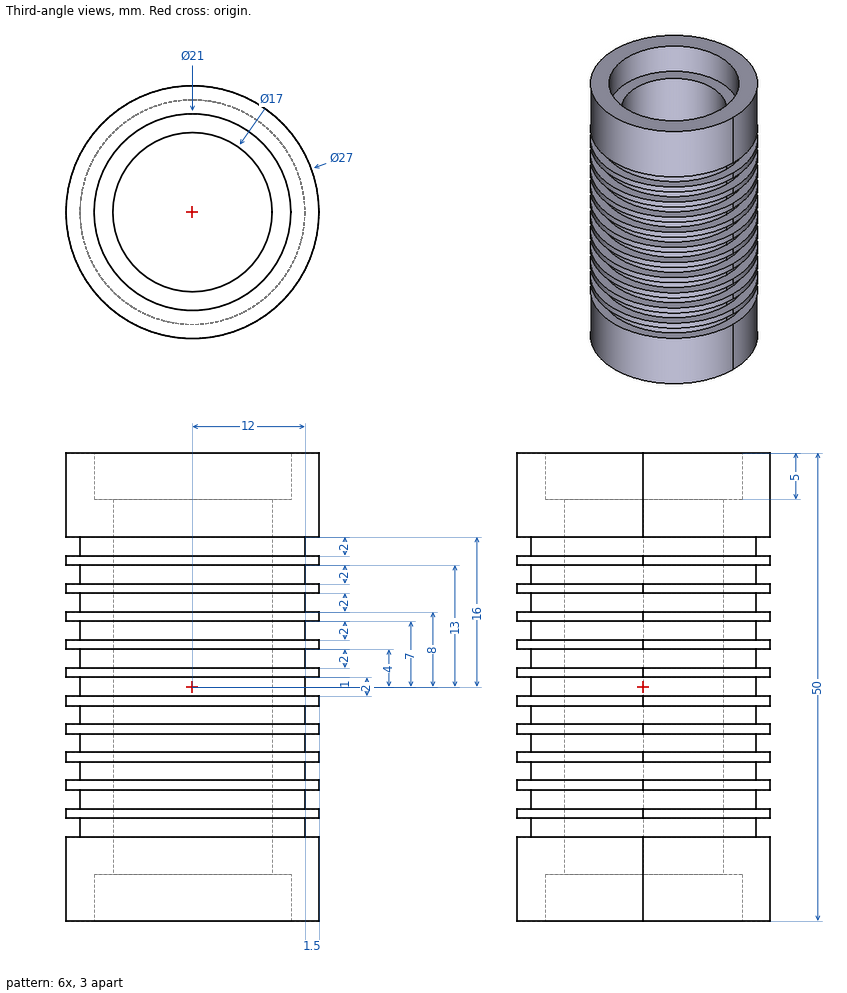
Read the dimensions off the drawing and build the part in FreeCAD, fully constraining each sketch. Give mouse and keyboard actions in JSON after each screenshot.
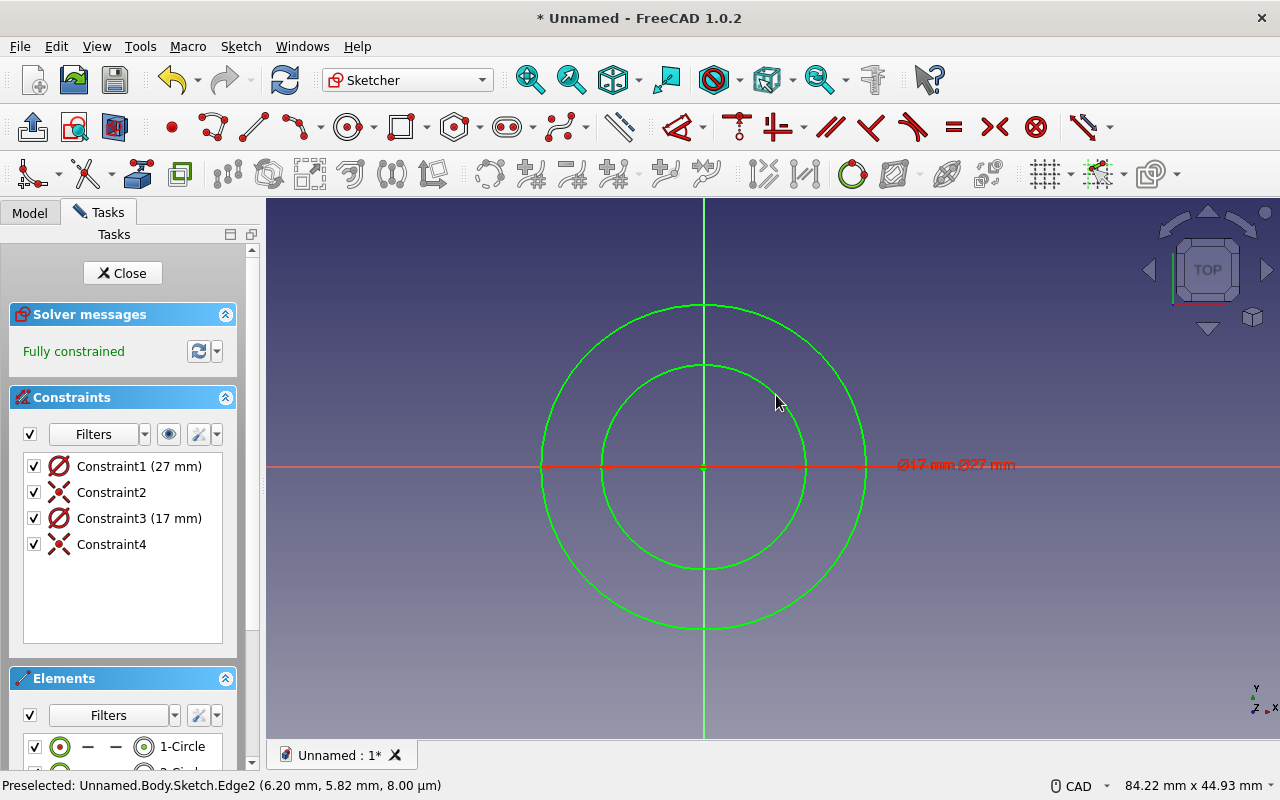
{"action": "left_click", "coordinate": [123, 273]}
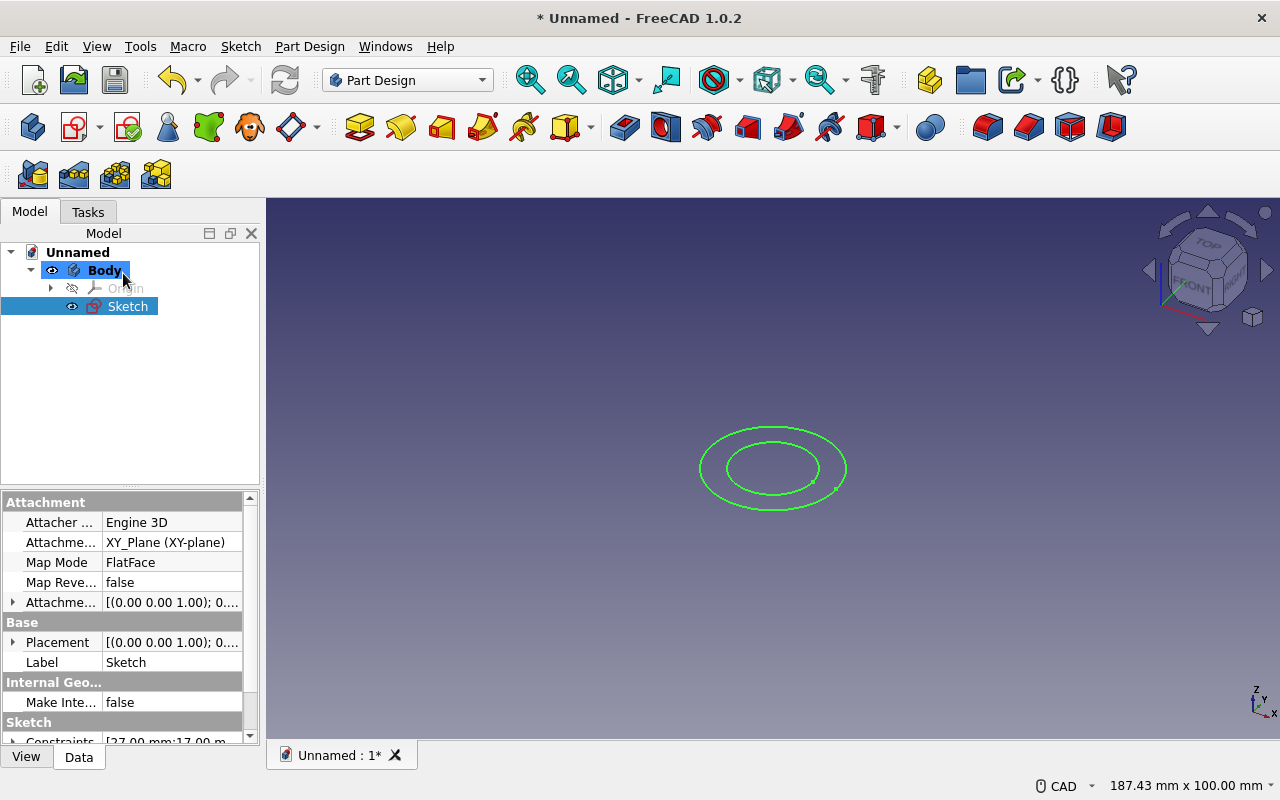
{"action": "left_click", "coordinate": [360, 128]}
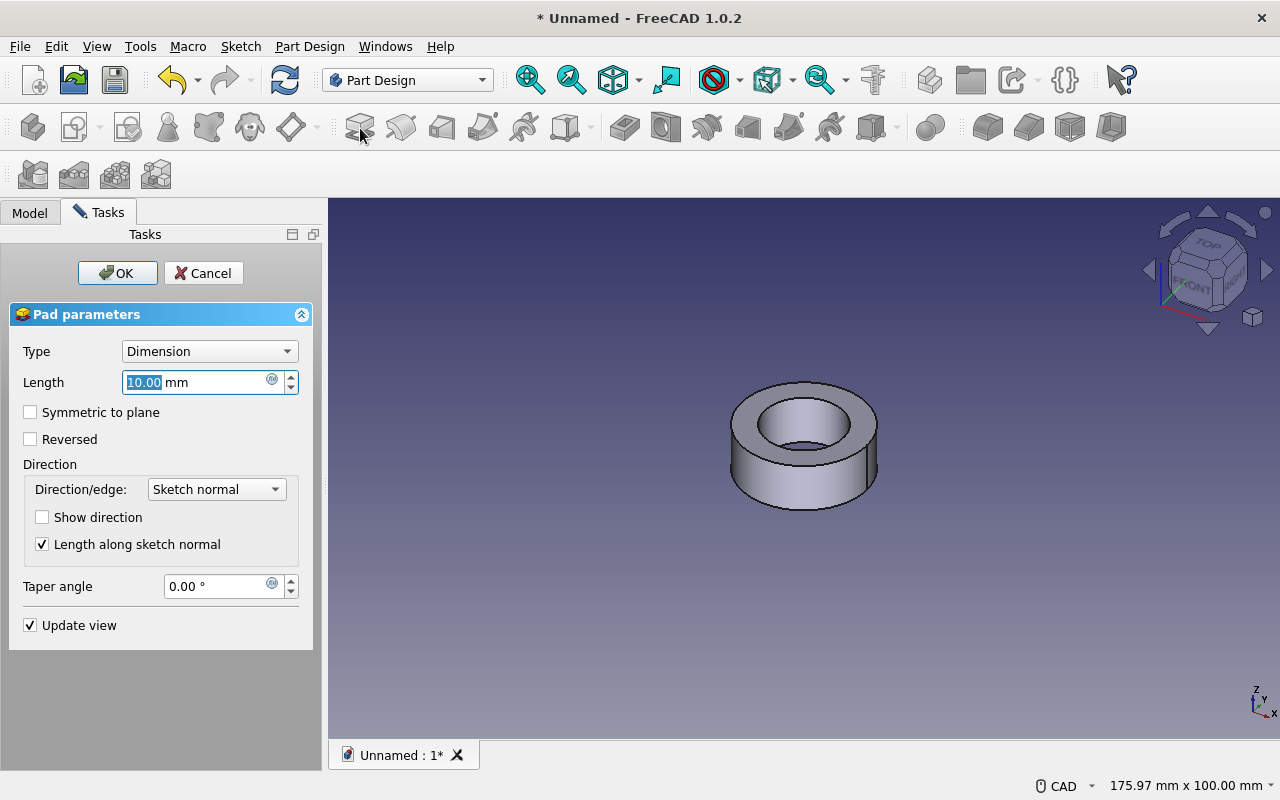
{"action": "type", "text": "50"}
{"action": "key", "text": "Tab"}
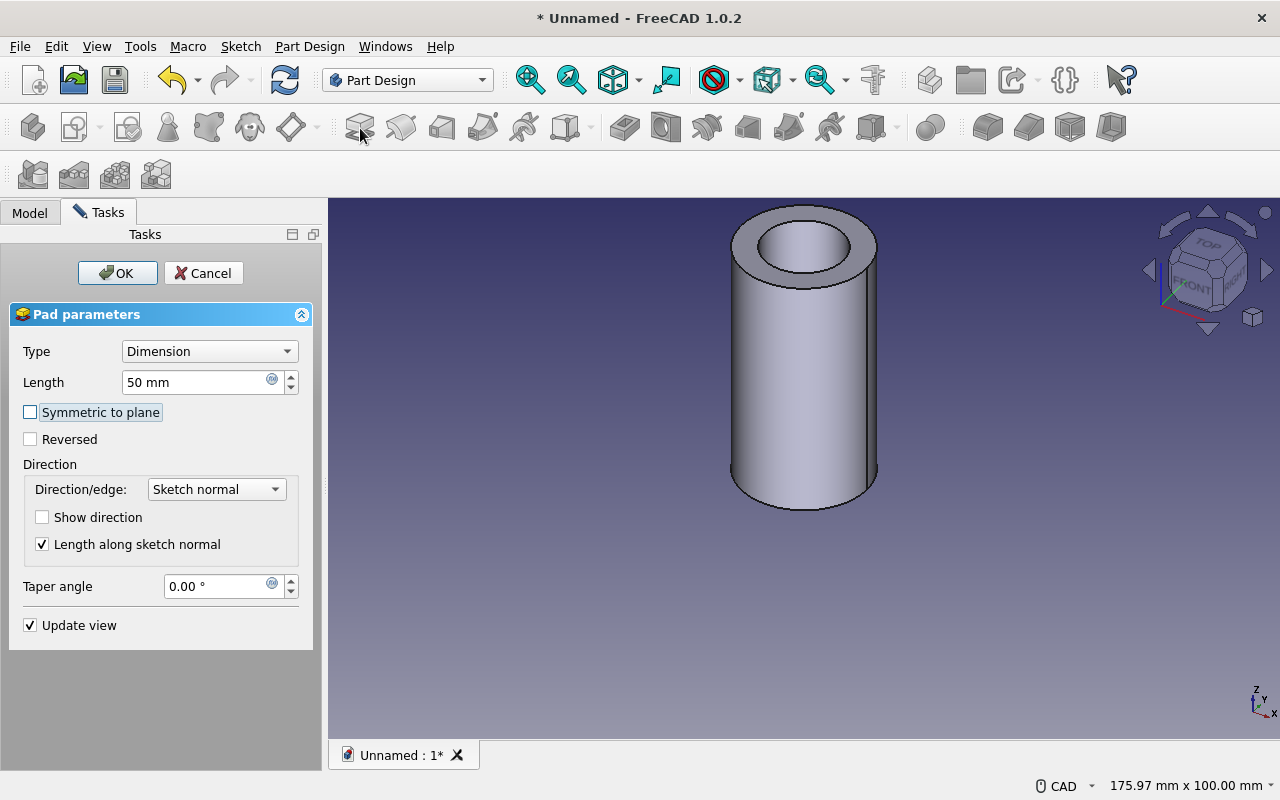
{"action": "left_click", "coordinate": [31, 412]}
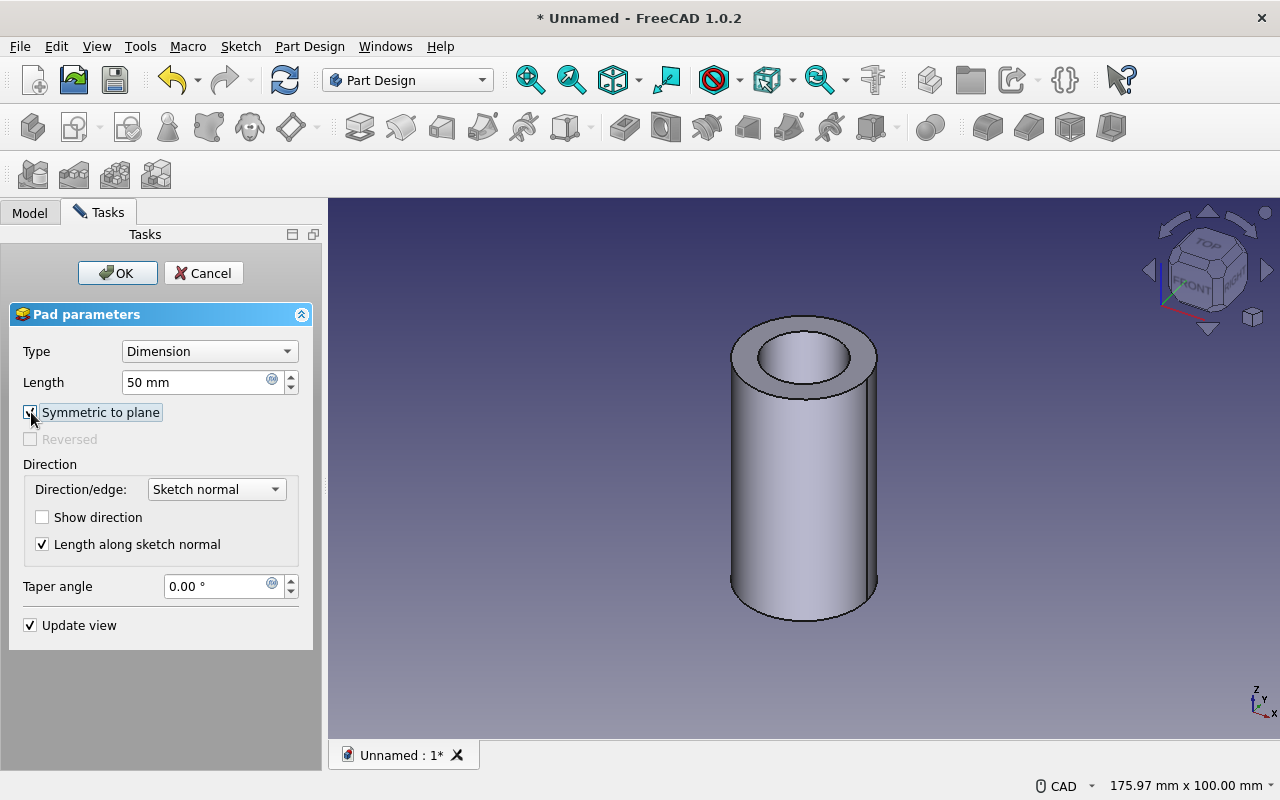
{"action": "left_click", "coordinate": [118, 273]}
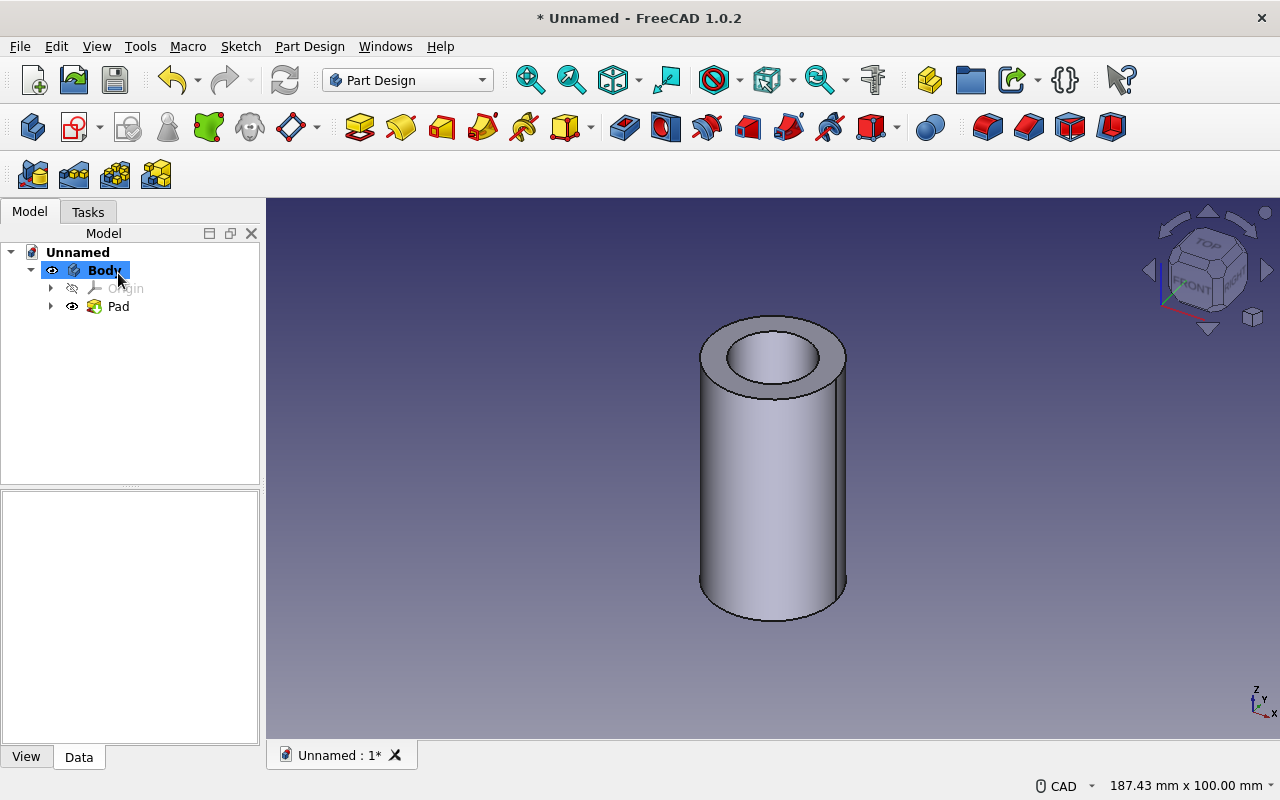
{"action": "left_click", "coordinate": [74, 128]}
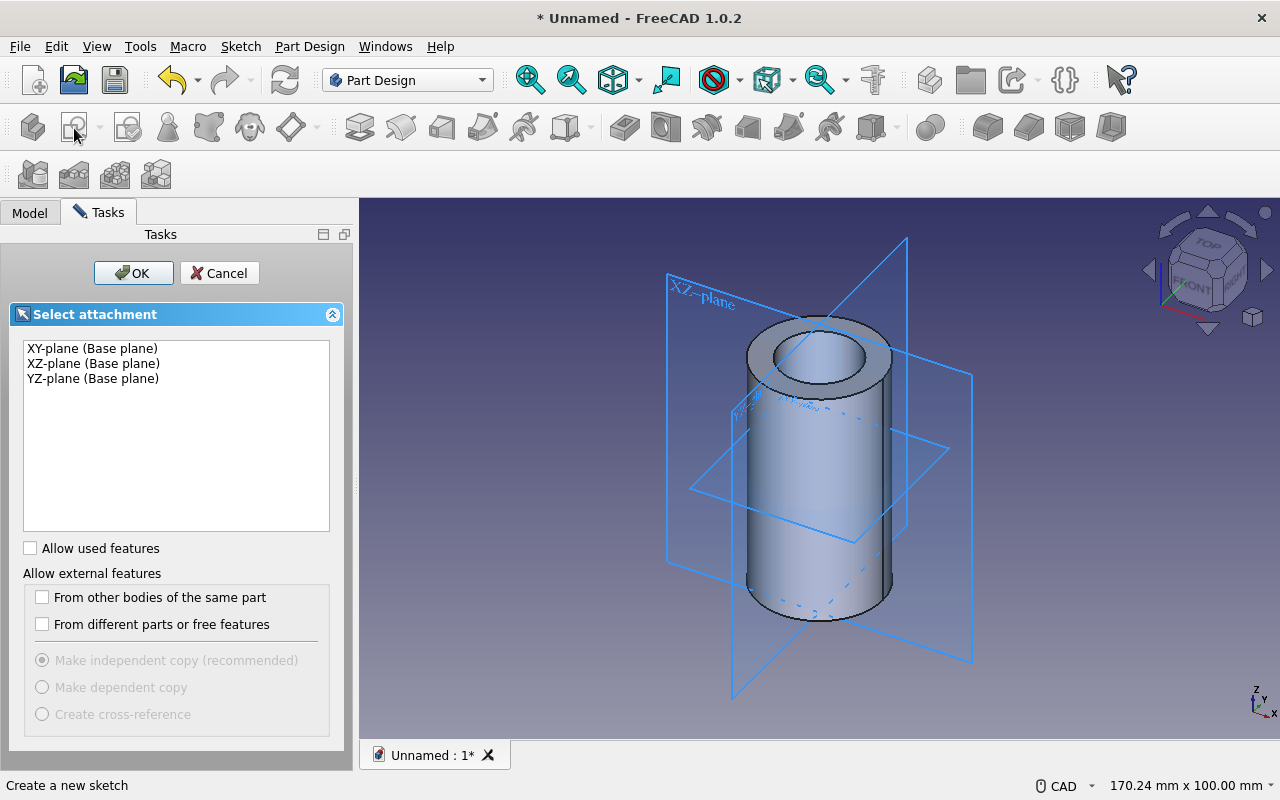
{"action": "left_click", "coordinate": [84, 364]}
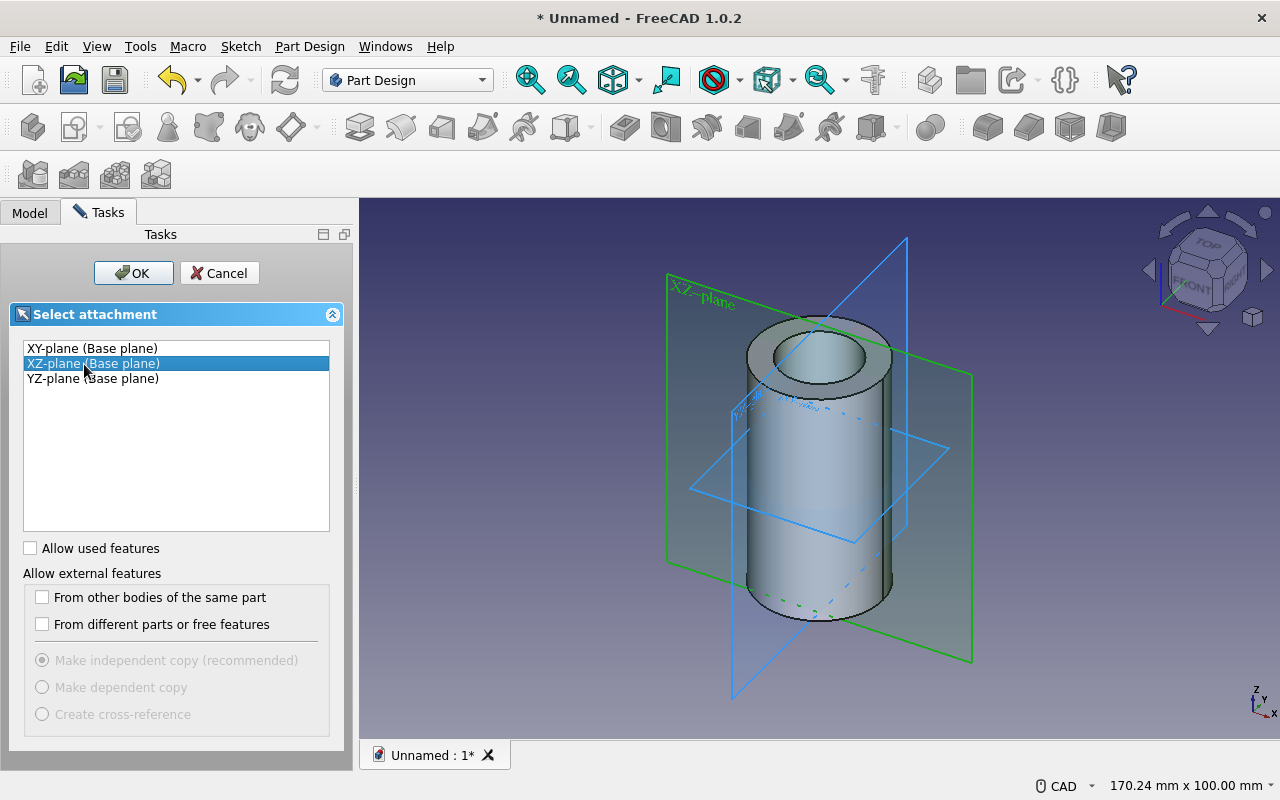
{"action": "left_click", "coordinate": [134, 273]}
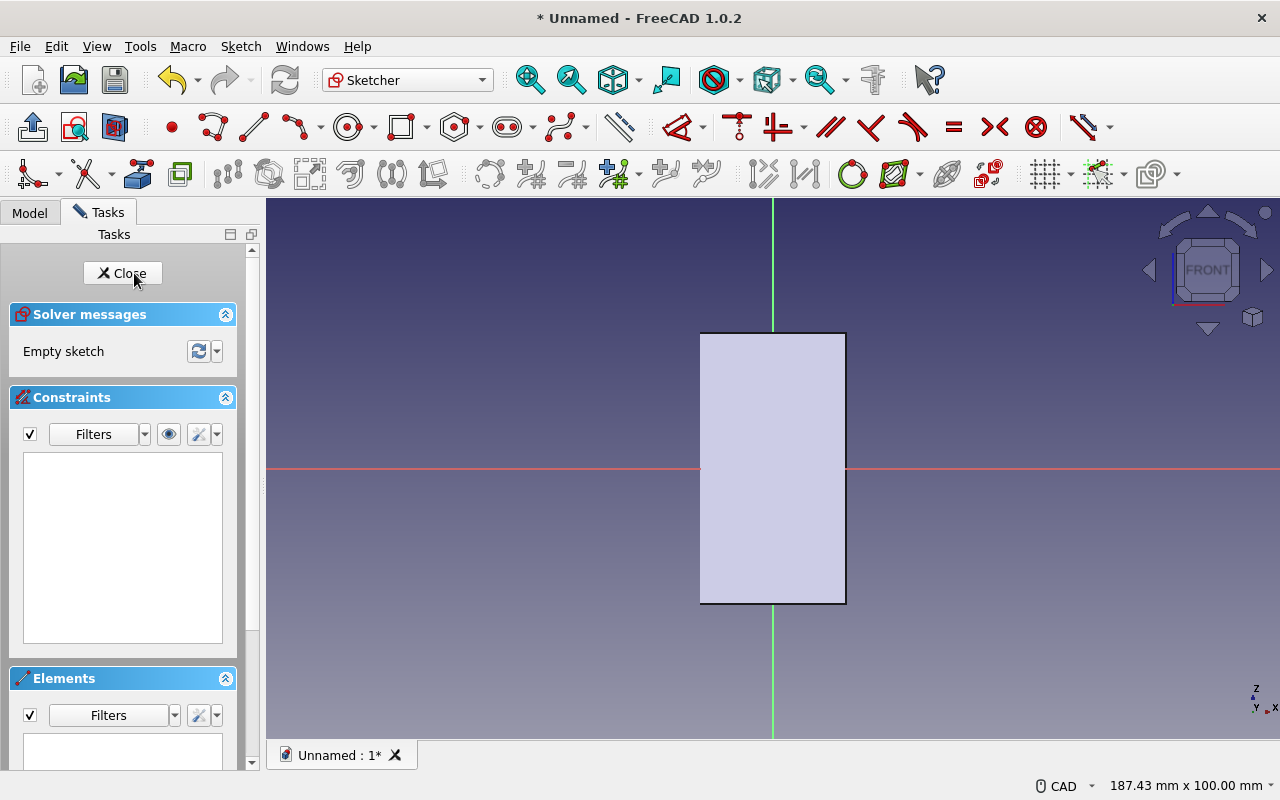
{"action": "left_click", "coordinate": [115, 128]}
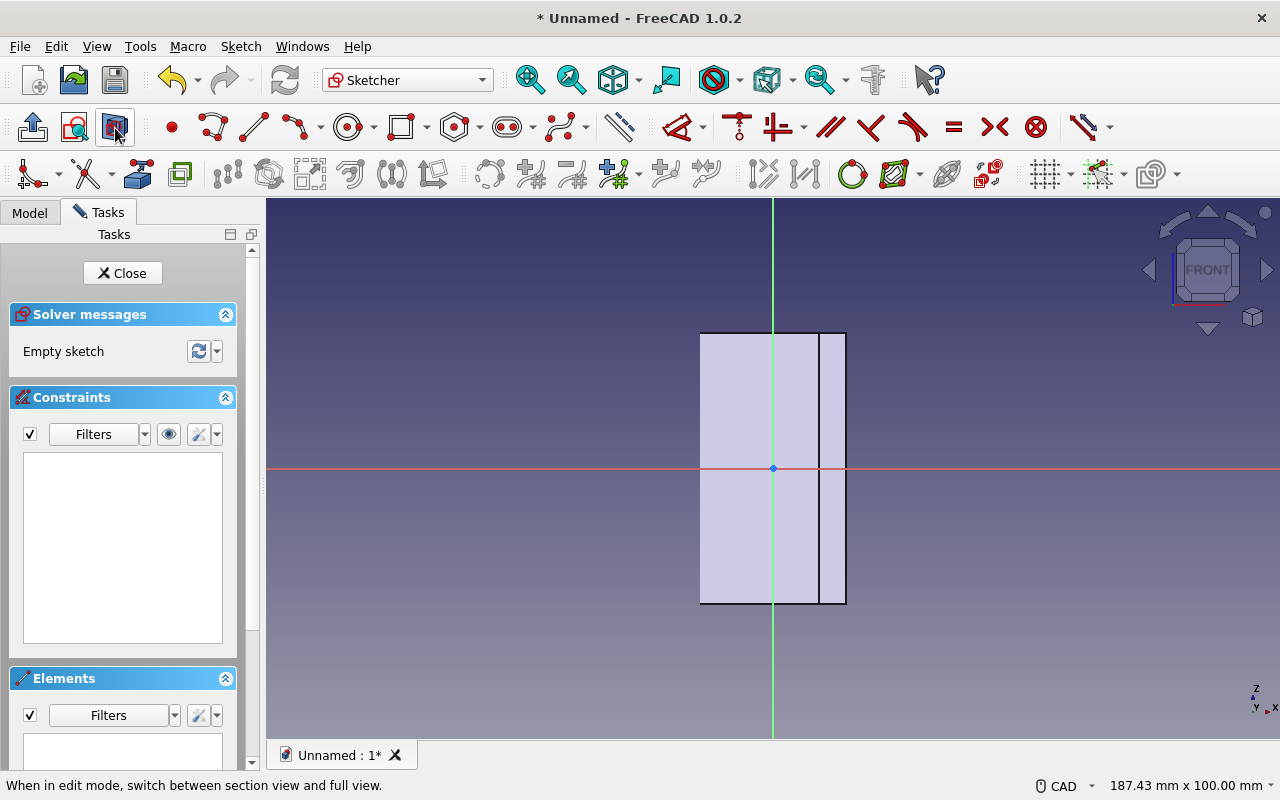
{"action": "scroll", "coordinate": [849, 468], "scroll_direction": "up", "scroll_amount": 15}